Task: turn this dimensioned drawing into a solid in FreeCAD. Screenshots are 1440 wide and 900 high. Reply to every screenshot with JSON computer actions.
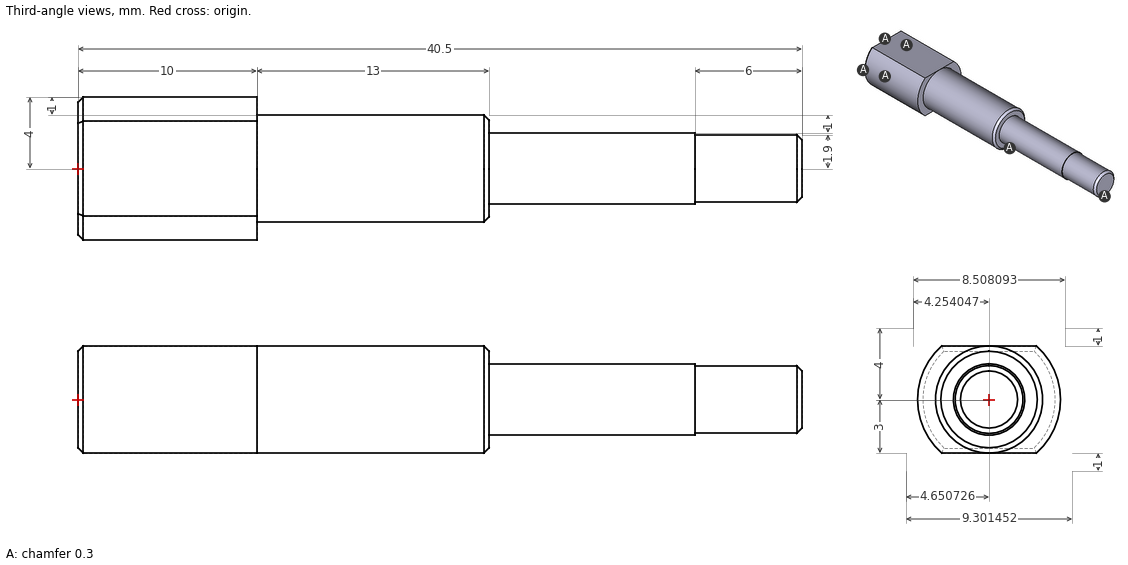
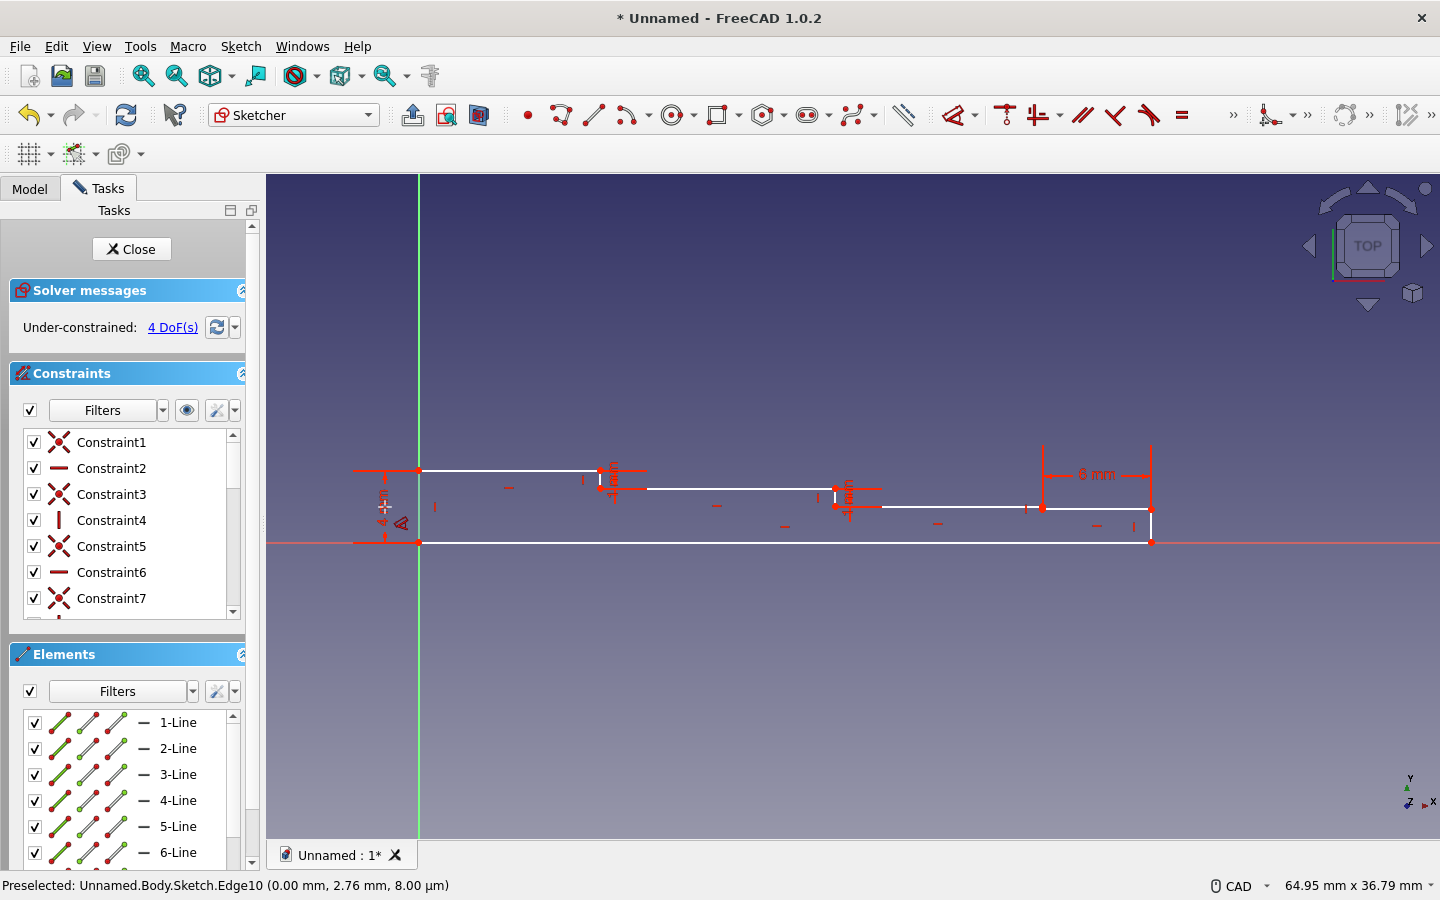
{"action": "left_click", "coordinate": [764, 489]}
{"action": "left_click", "coordinate": [717, 455]}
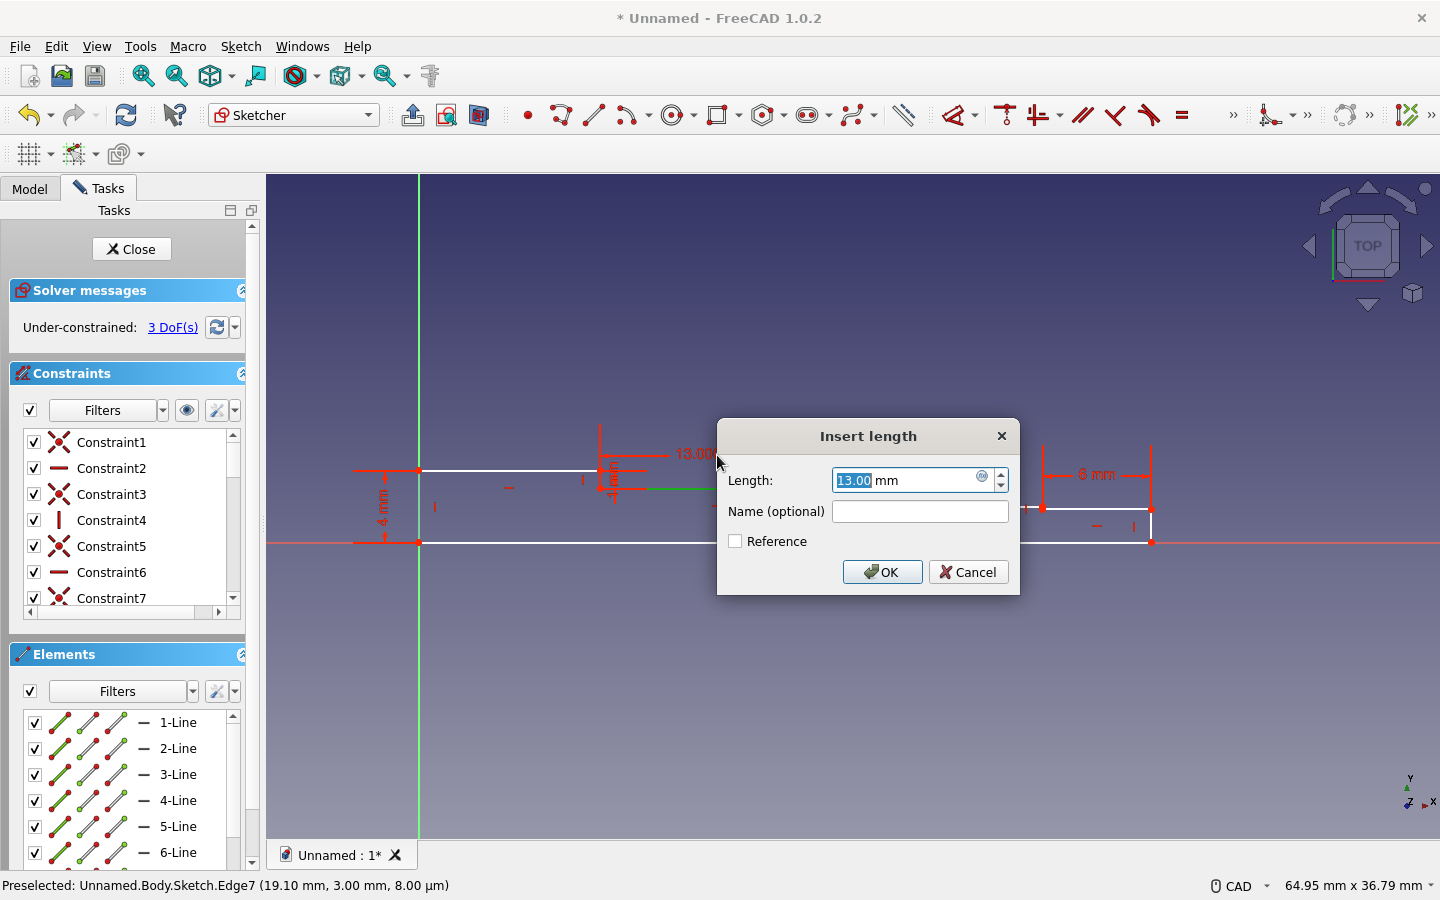
{"action": "type", "text": "13"}
{"action": "key", "text": "Return"}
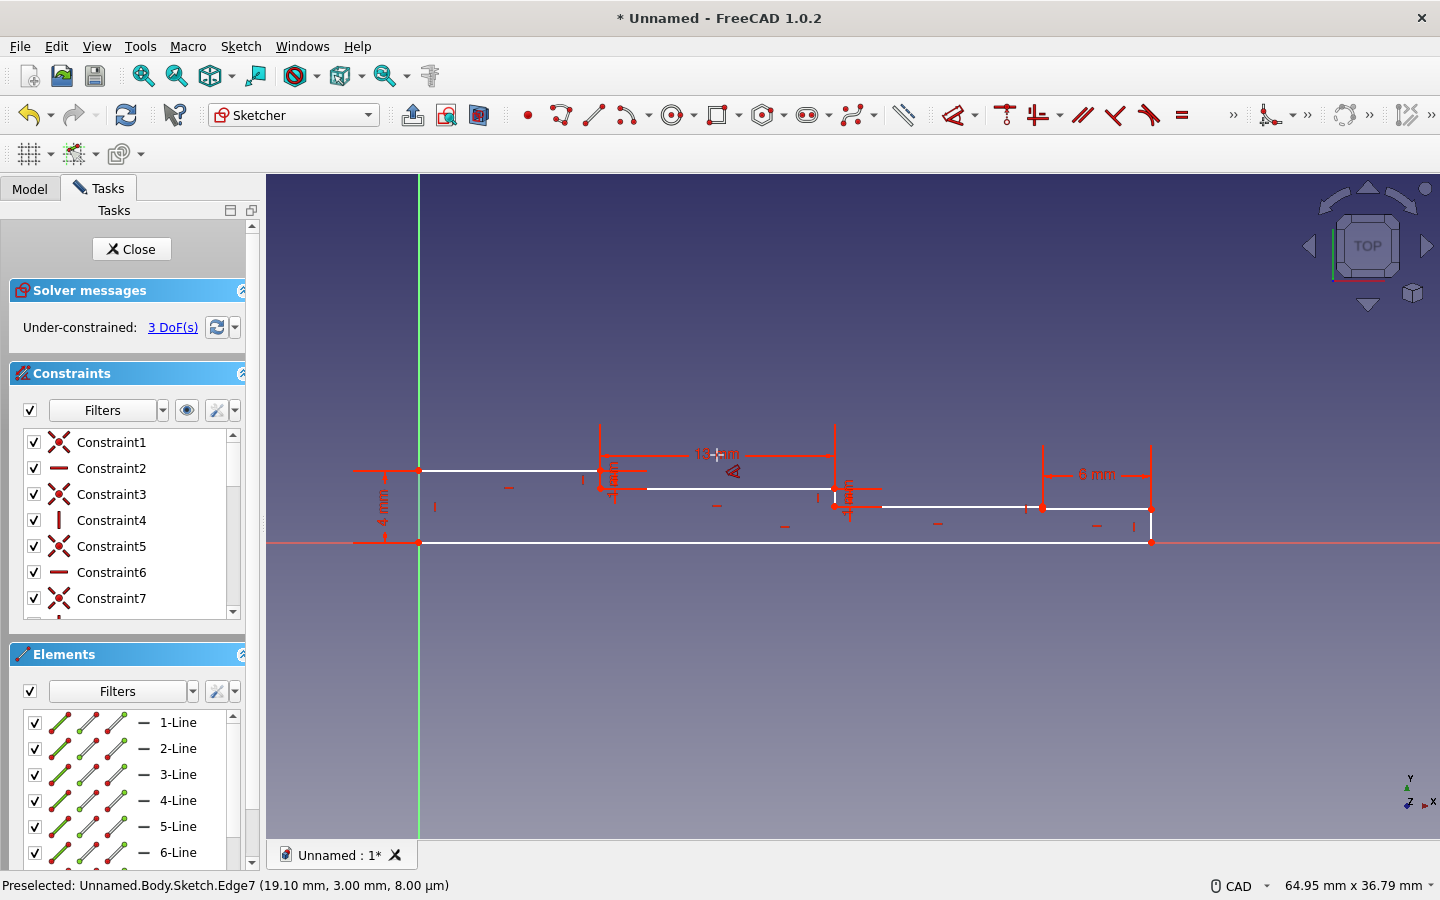
{"action": "left_click", "coordinate": [546, 471]}
{"action": "left_click", "coordinate": [509, 437]}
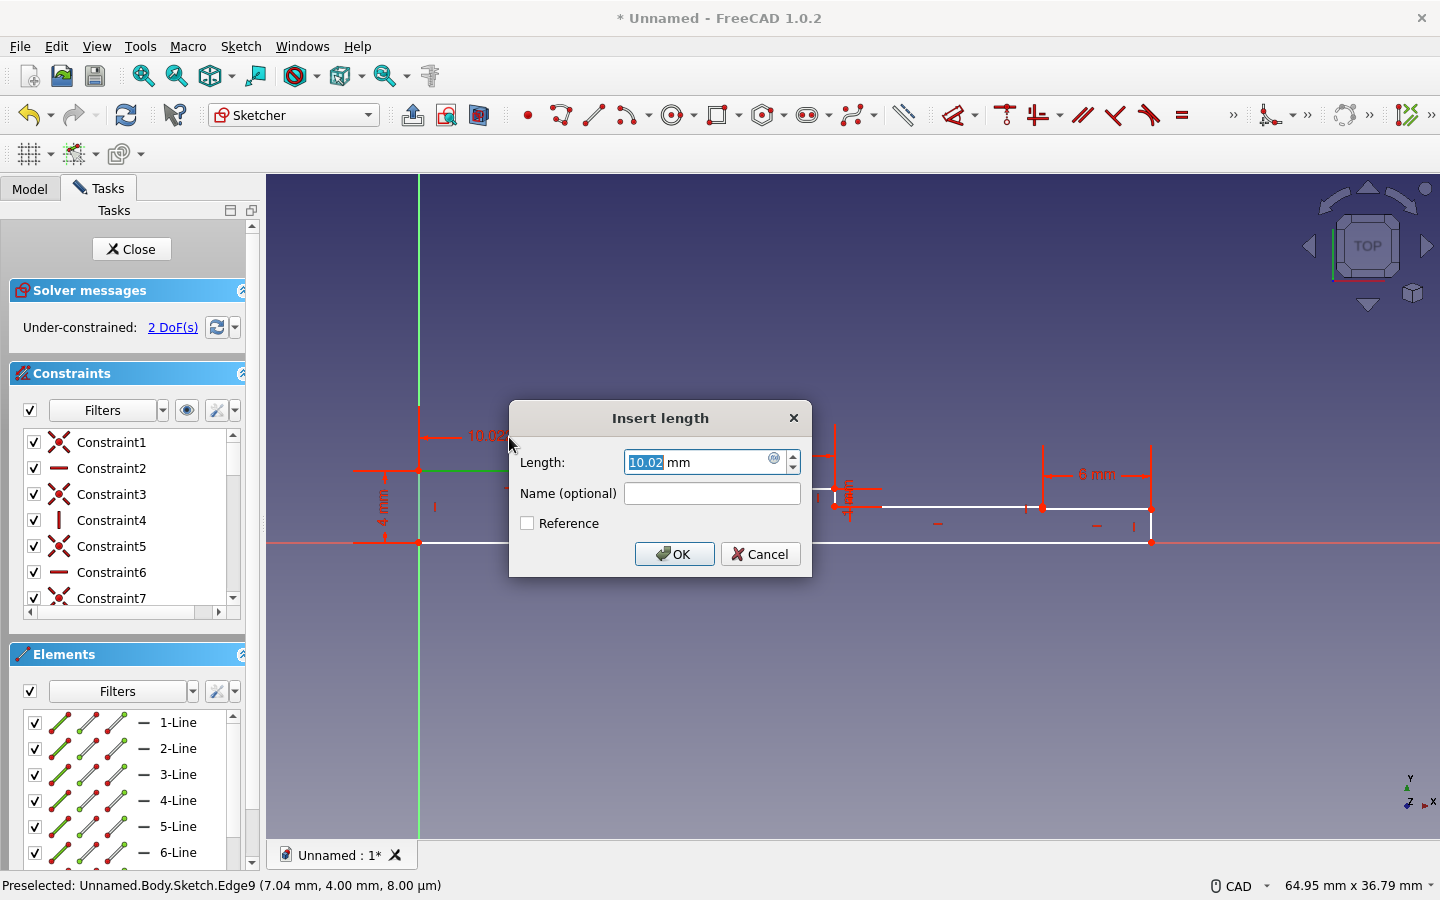
{"action": "type", "text": "10"}
{"action": "key", "text": "Return"}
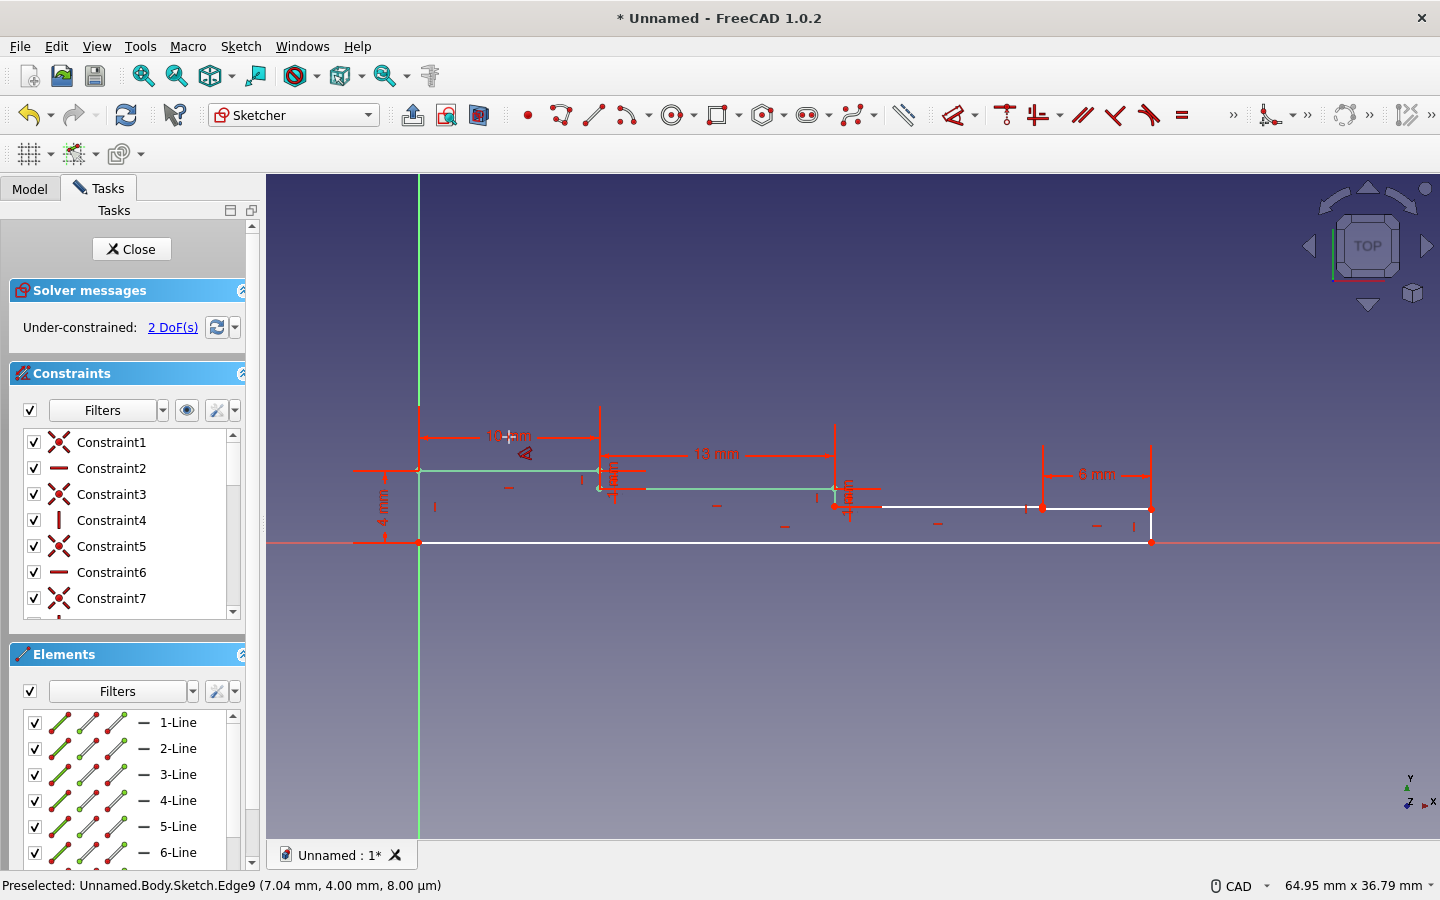
{"action": "scroll", "coordinate": [1151, 533], "scroll_direction": "up", "scroll_amount": 2}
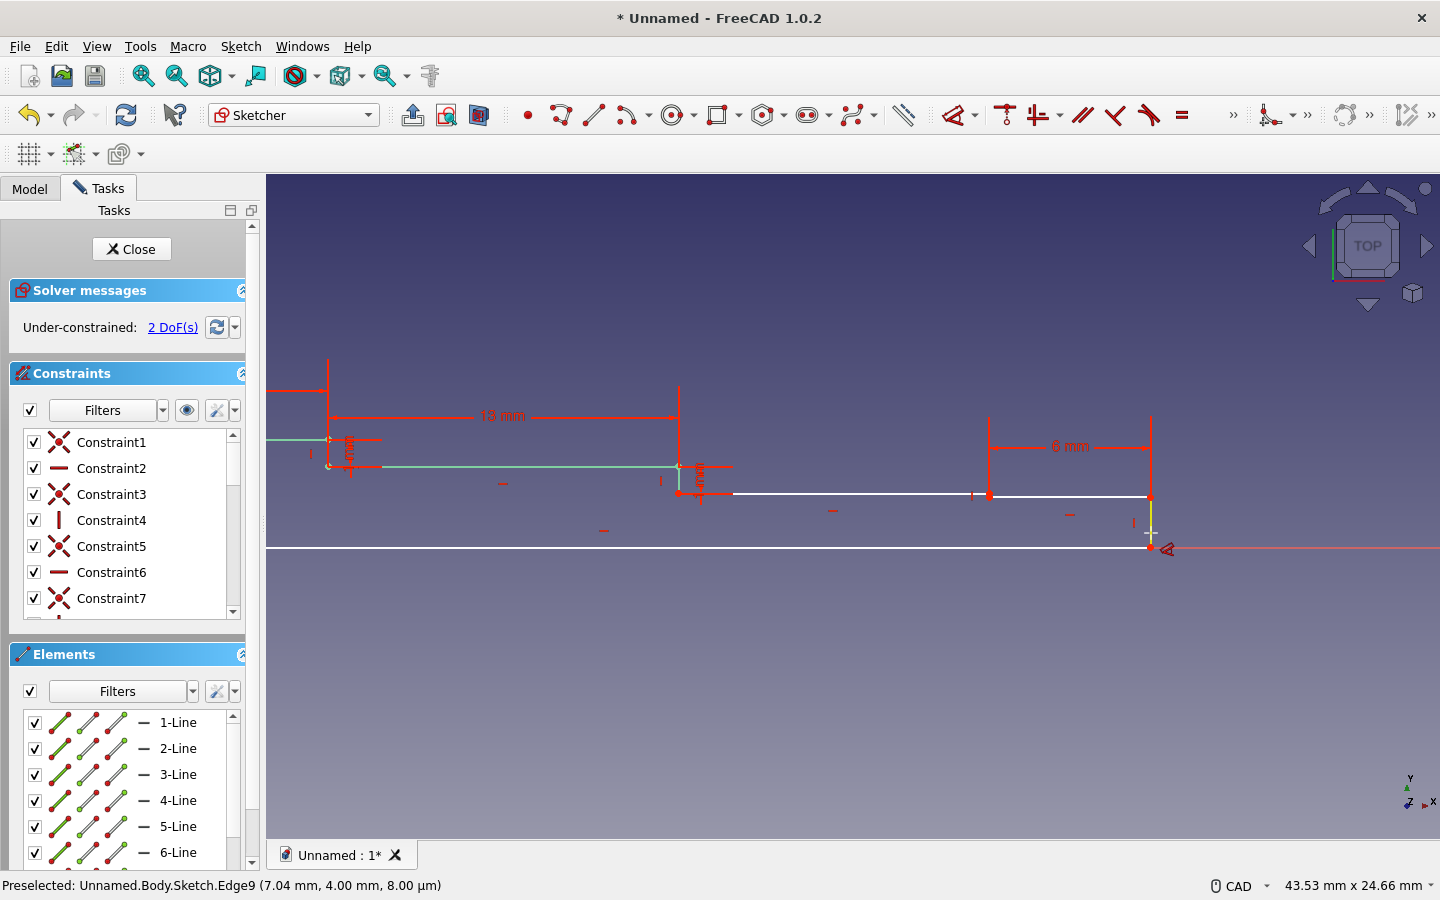
{"action": "left_click", "coordinate": [1151, 533]}
{"action": "left_click", "coordinate": [1185, 523]}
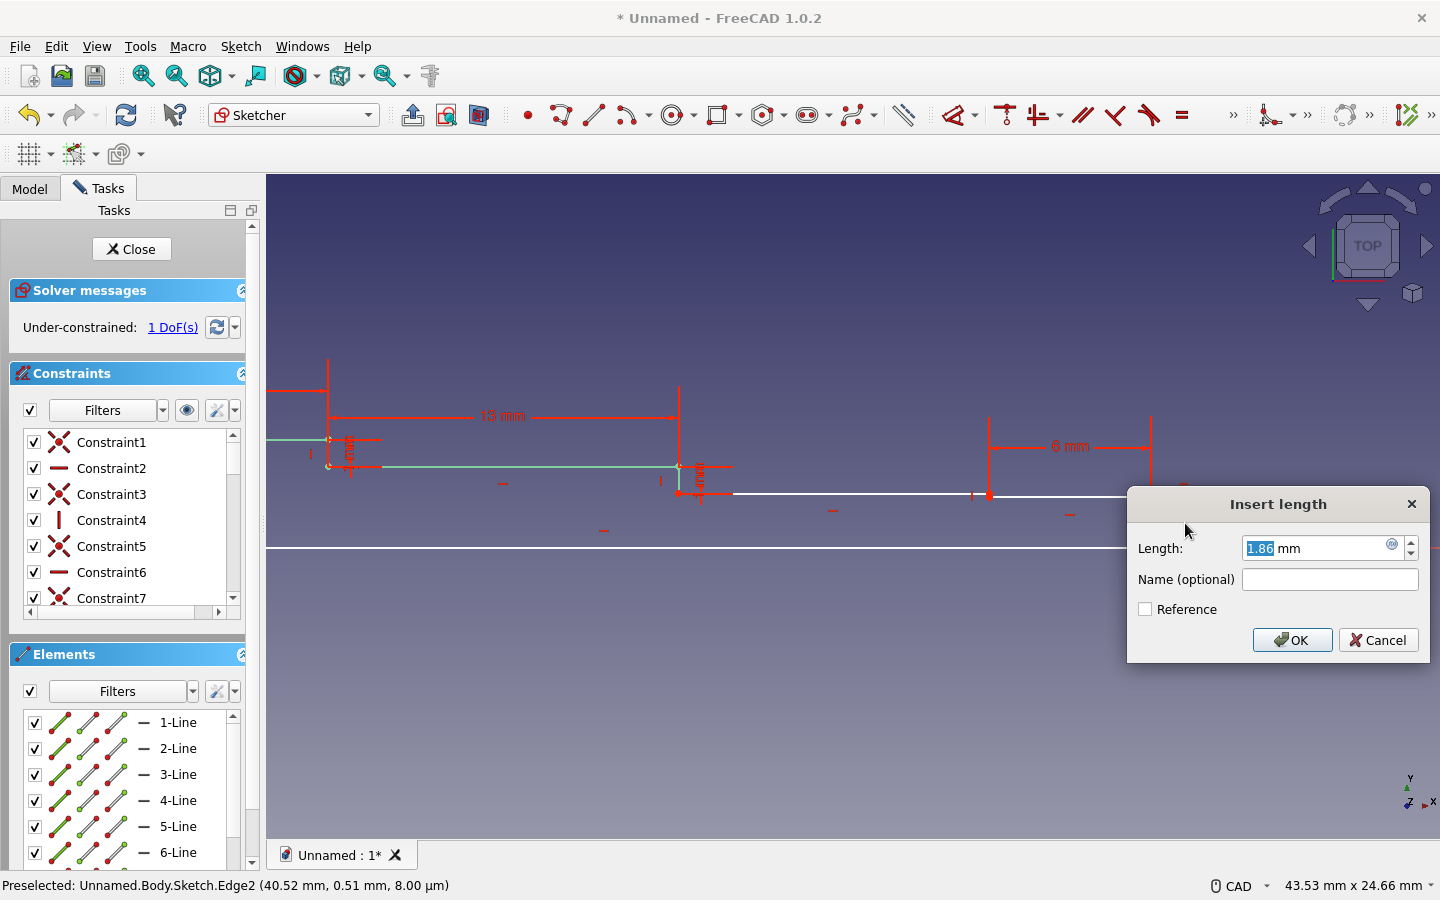
{"action": "type", "text": "1.9"}
{"action": "key", "text": "Return"}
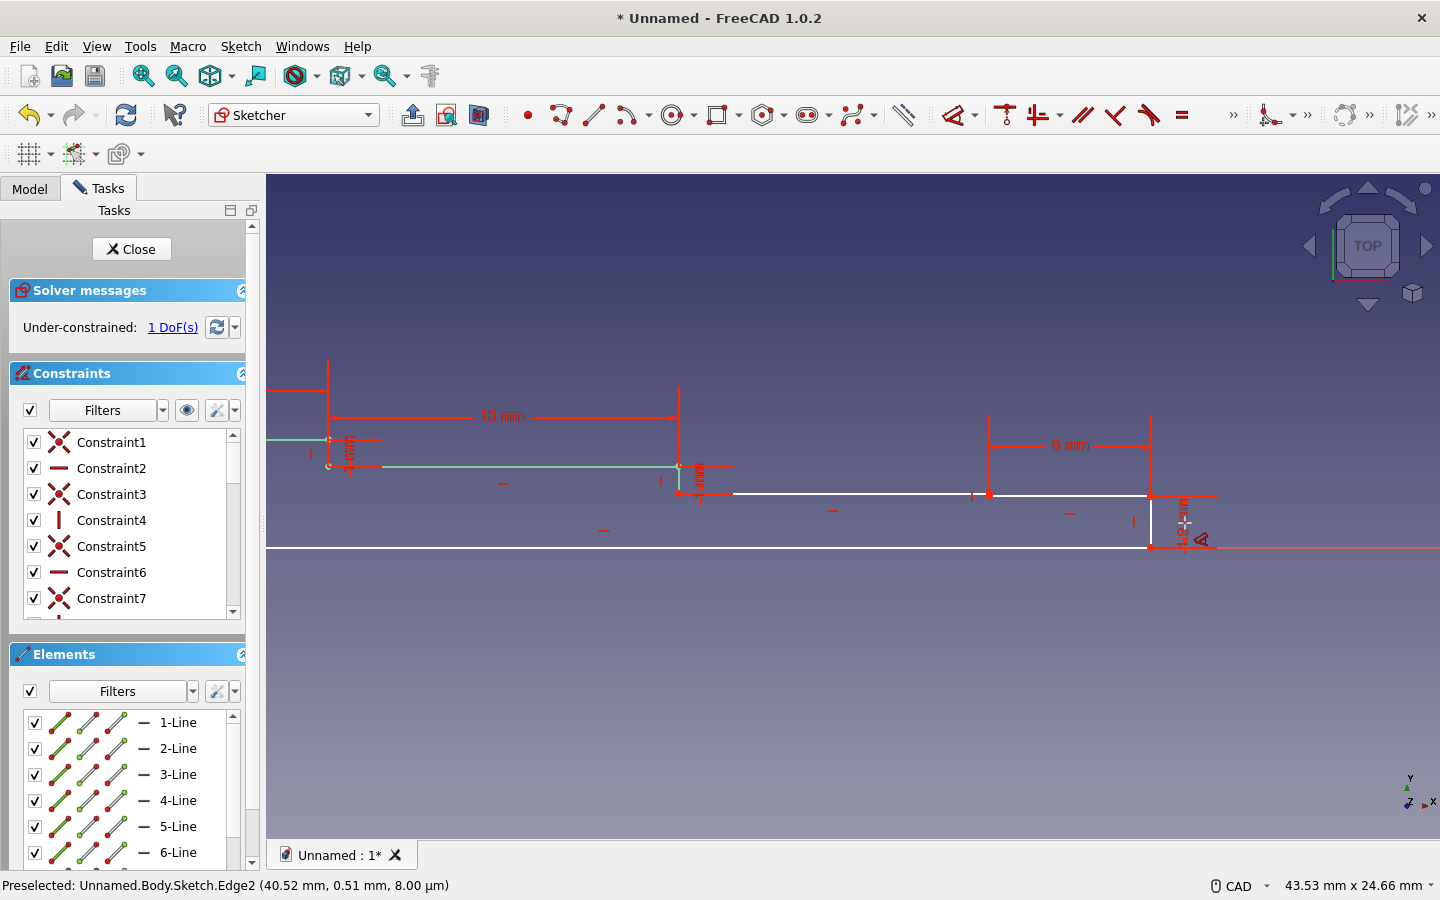
{"action": "left_click", "coordinate": [386, 548]}
{"action": "left_click", "coordinate": [722, 582]}